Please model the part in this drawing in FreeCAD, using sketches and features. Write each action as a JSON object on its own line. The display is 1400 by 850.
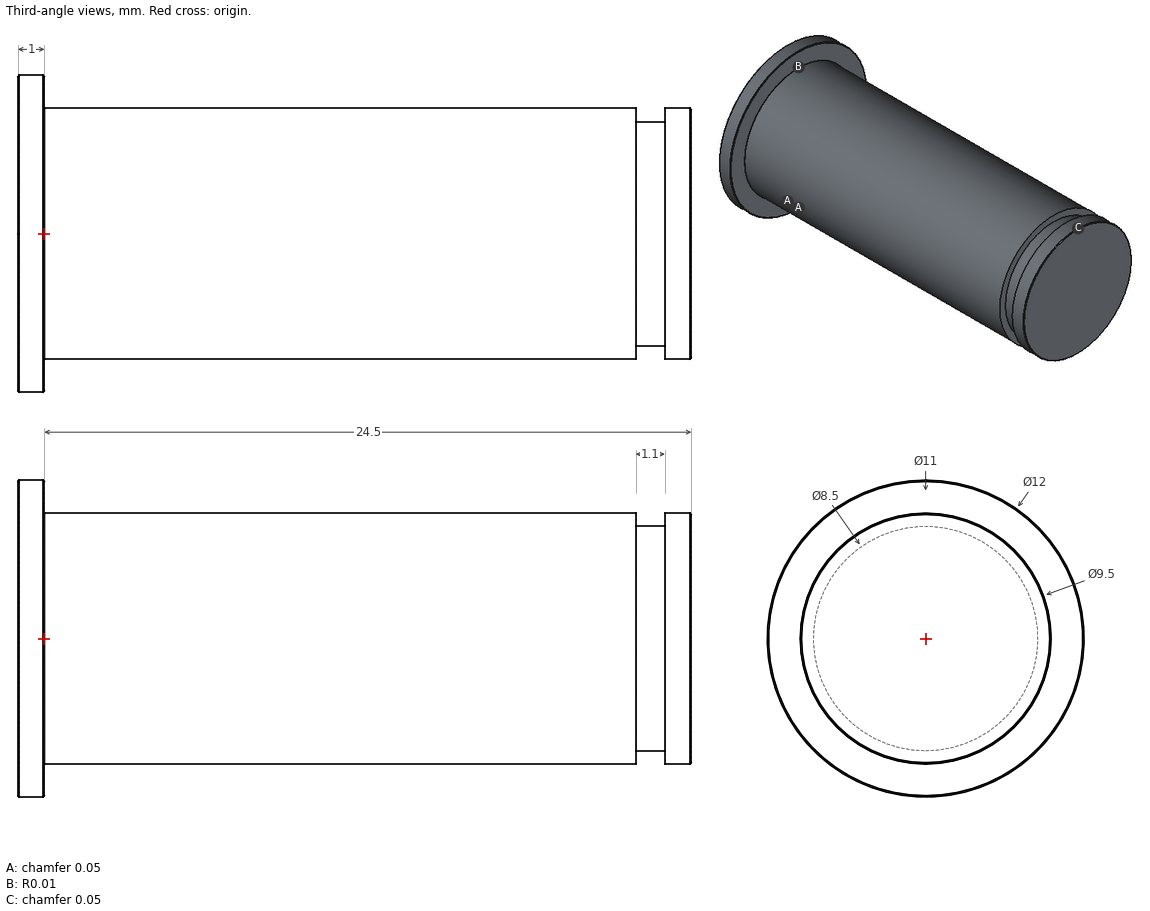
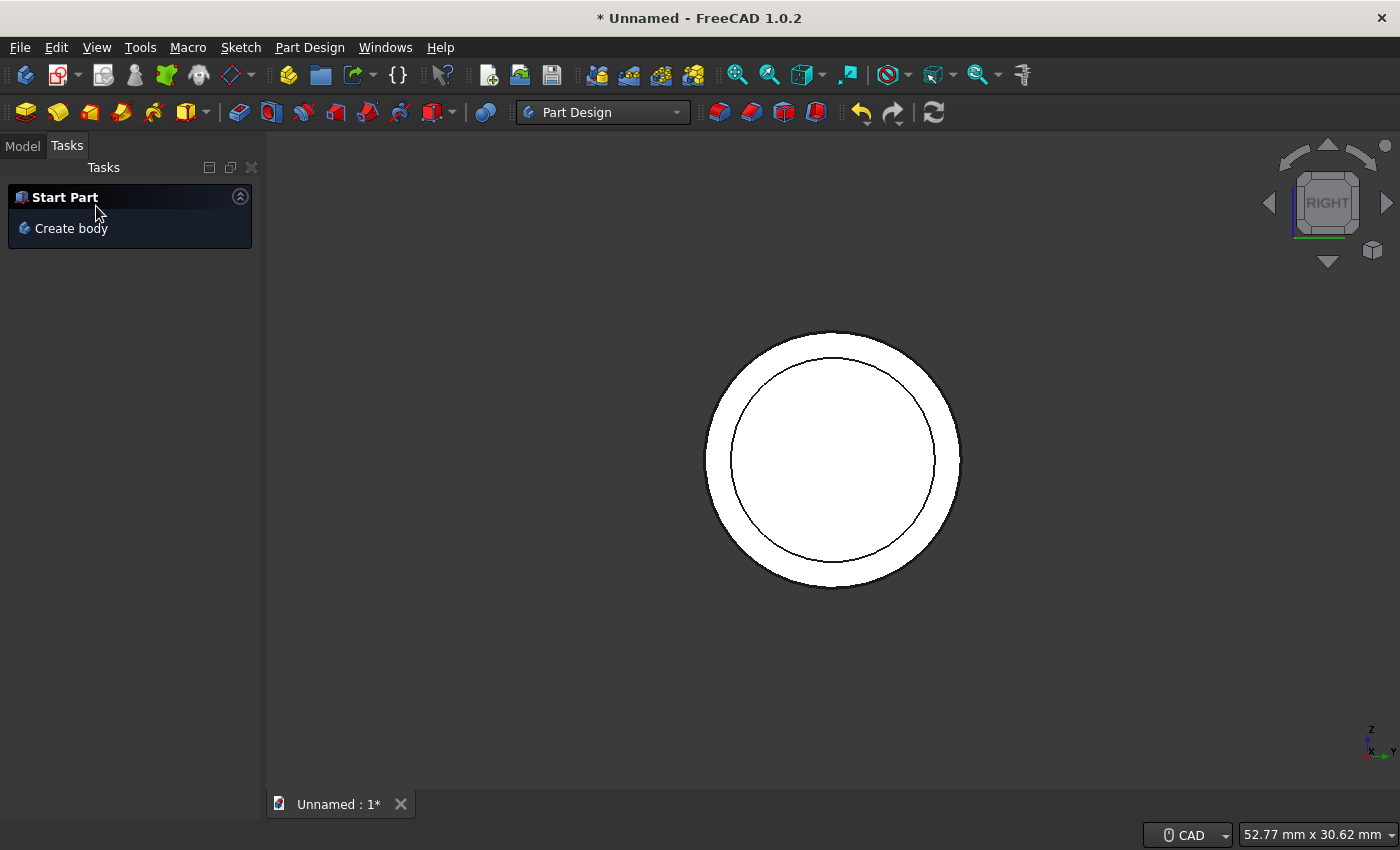
{"action": "key", "text": "v f"}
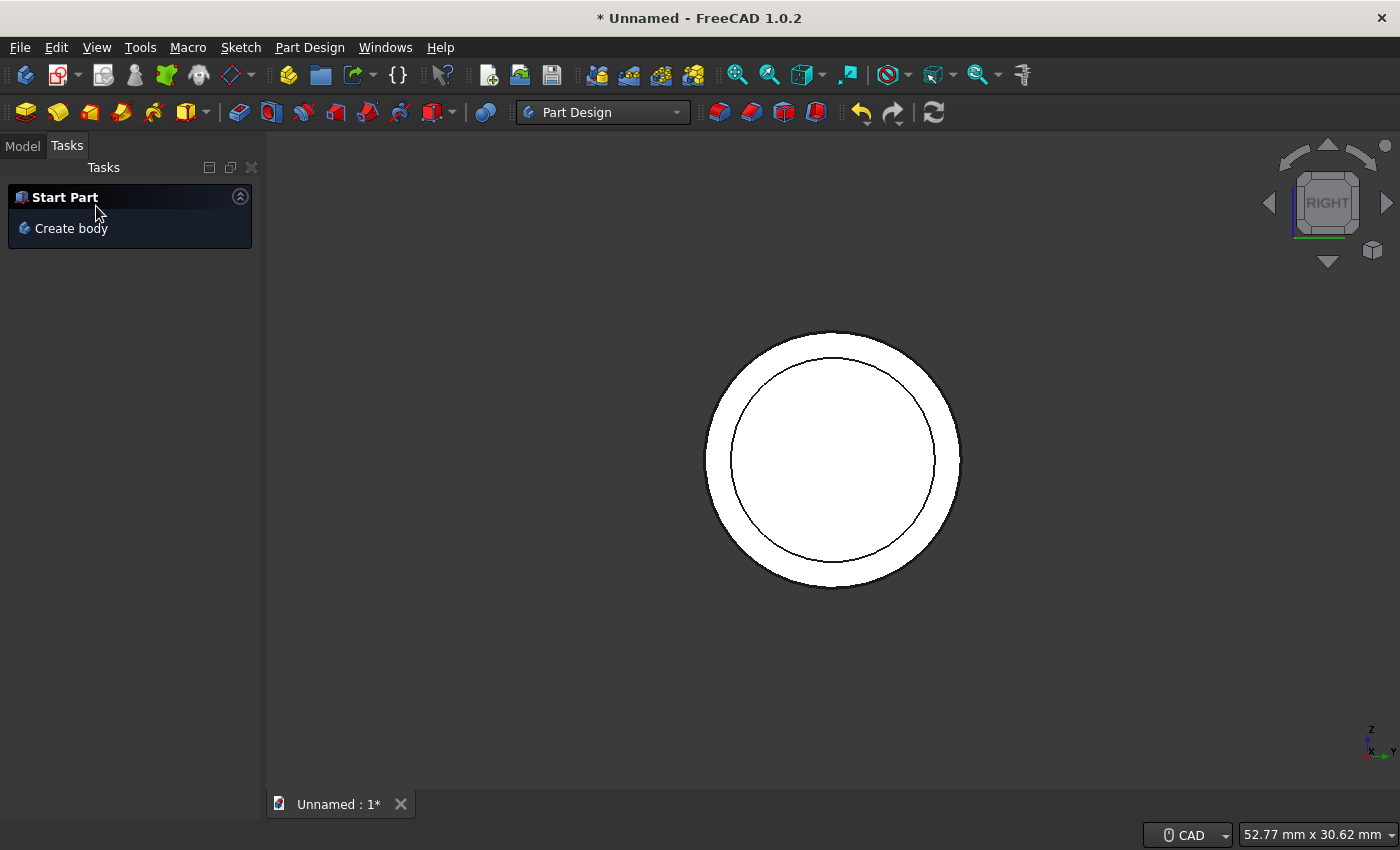
{"action": "key", "text": "5"}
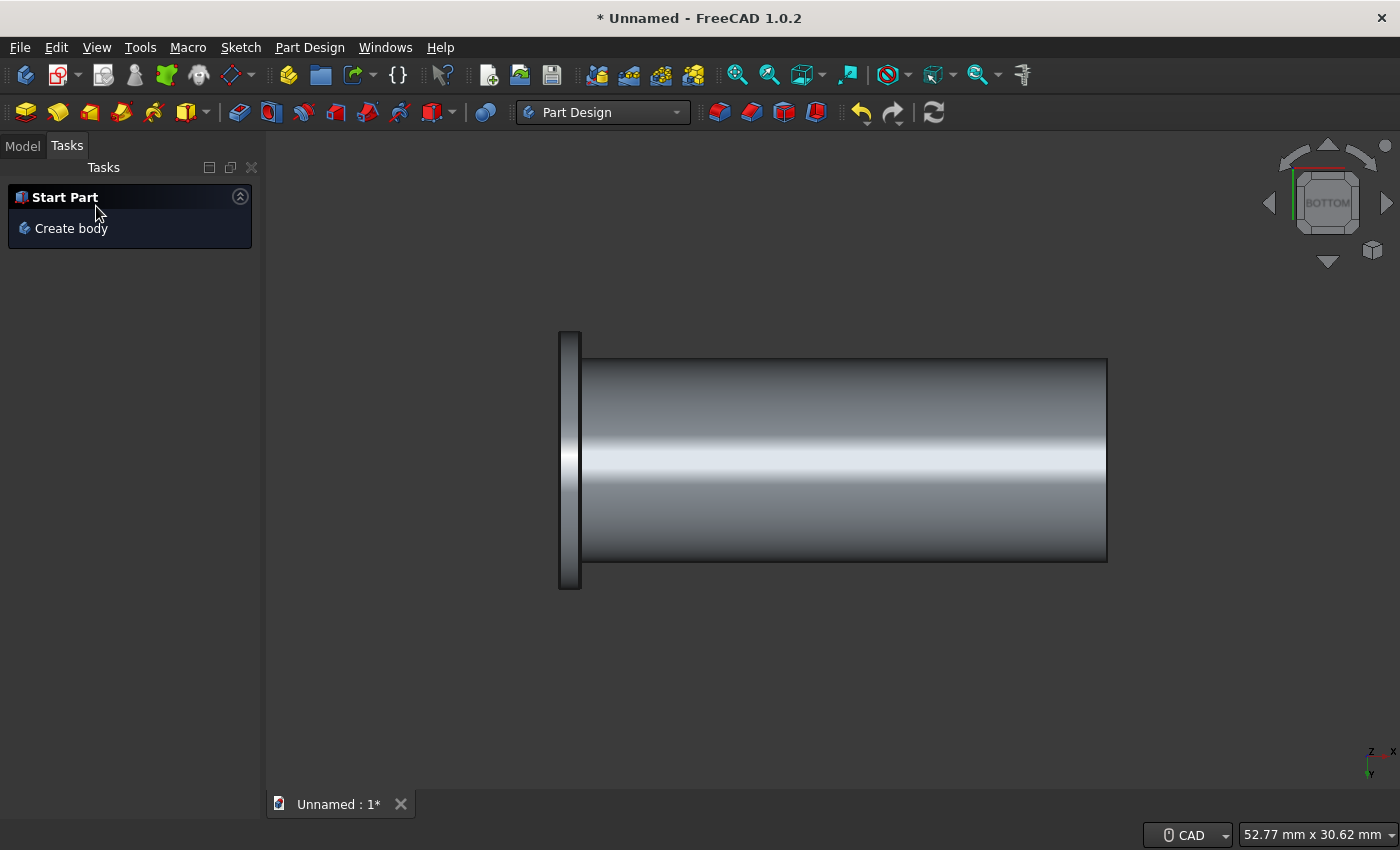
{"action": "key", "text": "4"}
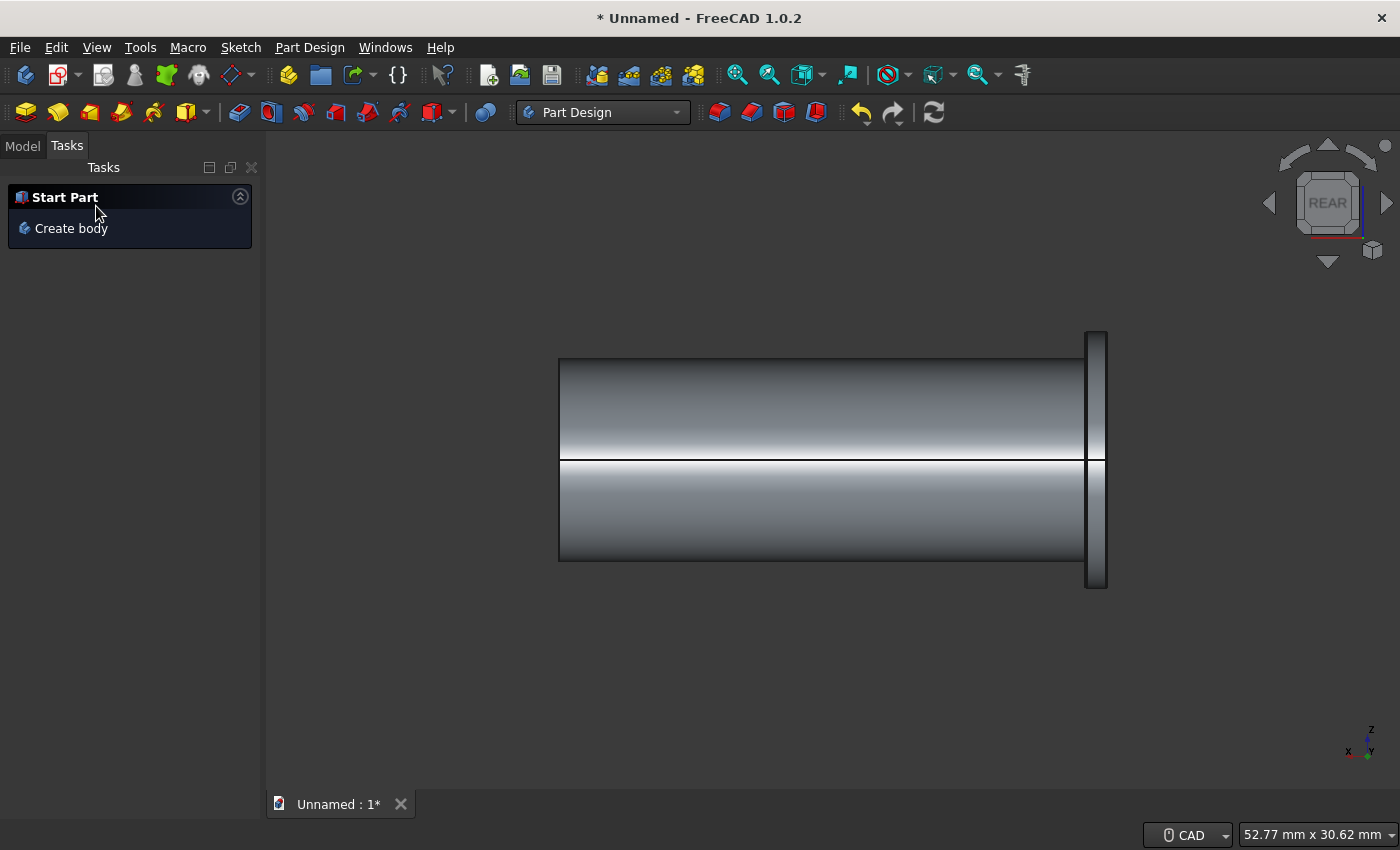
{"action": "key", "text": "6"}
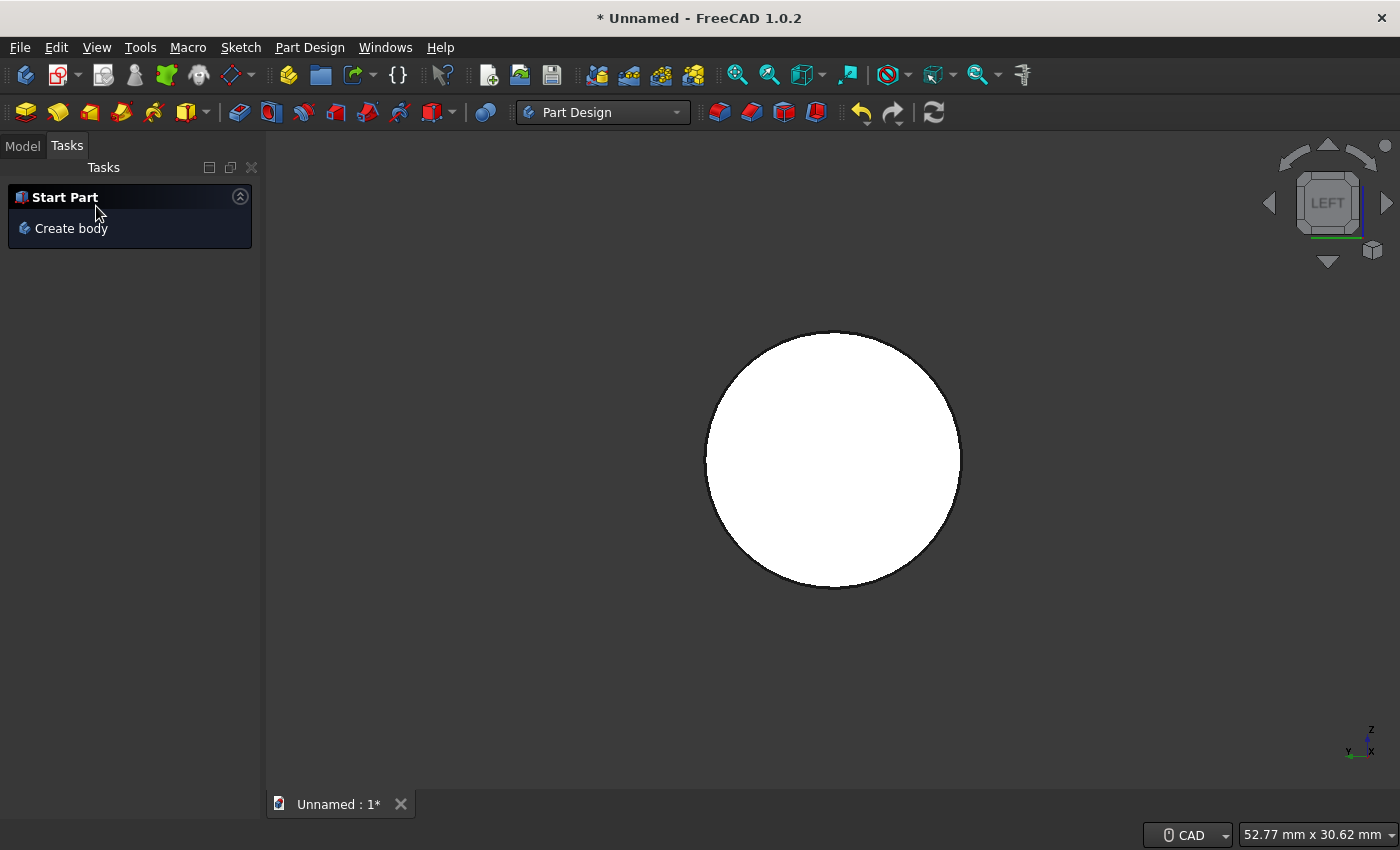
{"action": "key", "text": "v f"}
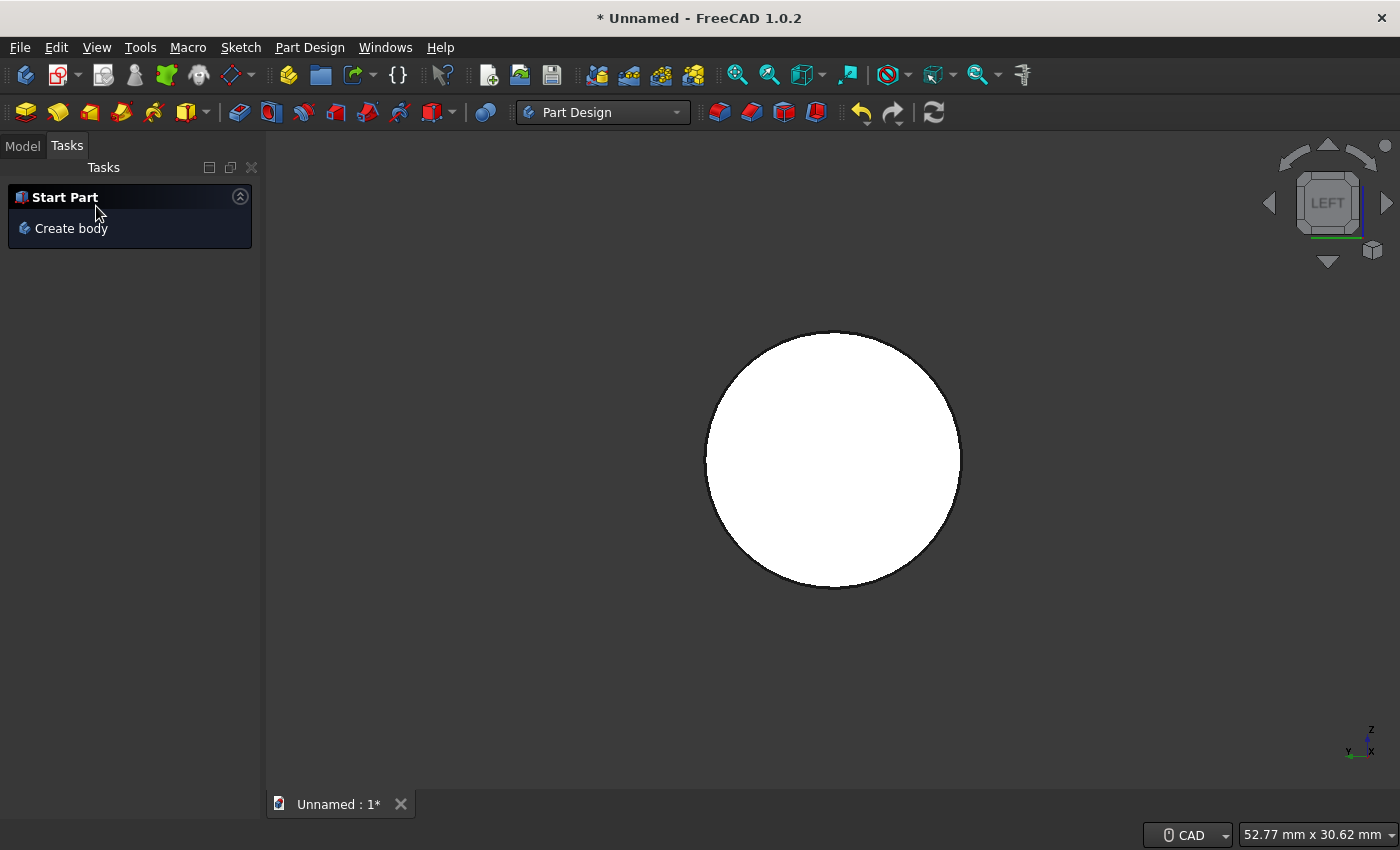
{"action": "key", "text": "v 3"}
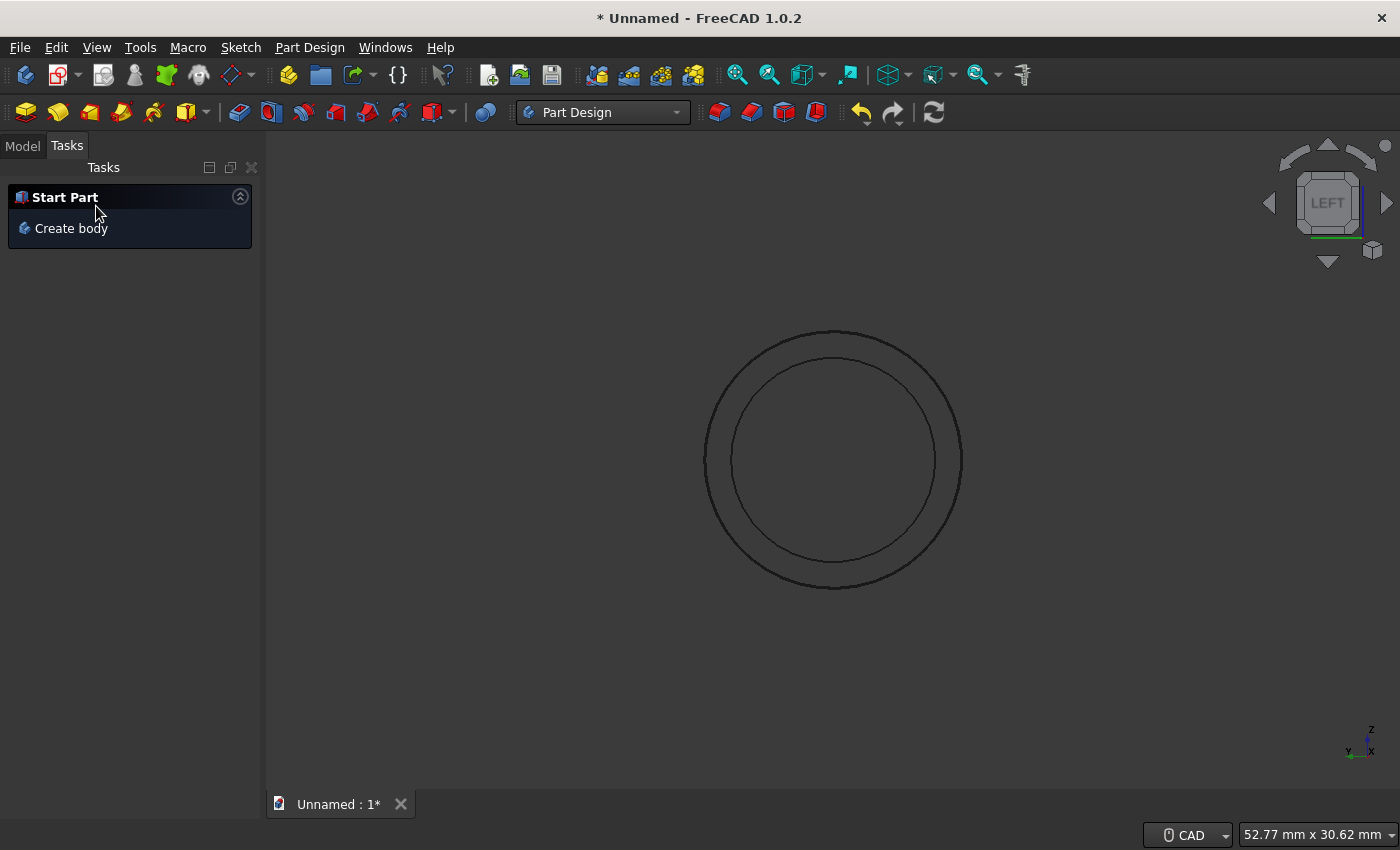
{"action": "key", "text": "0"}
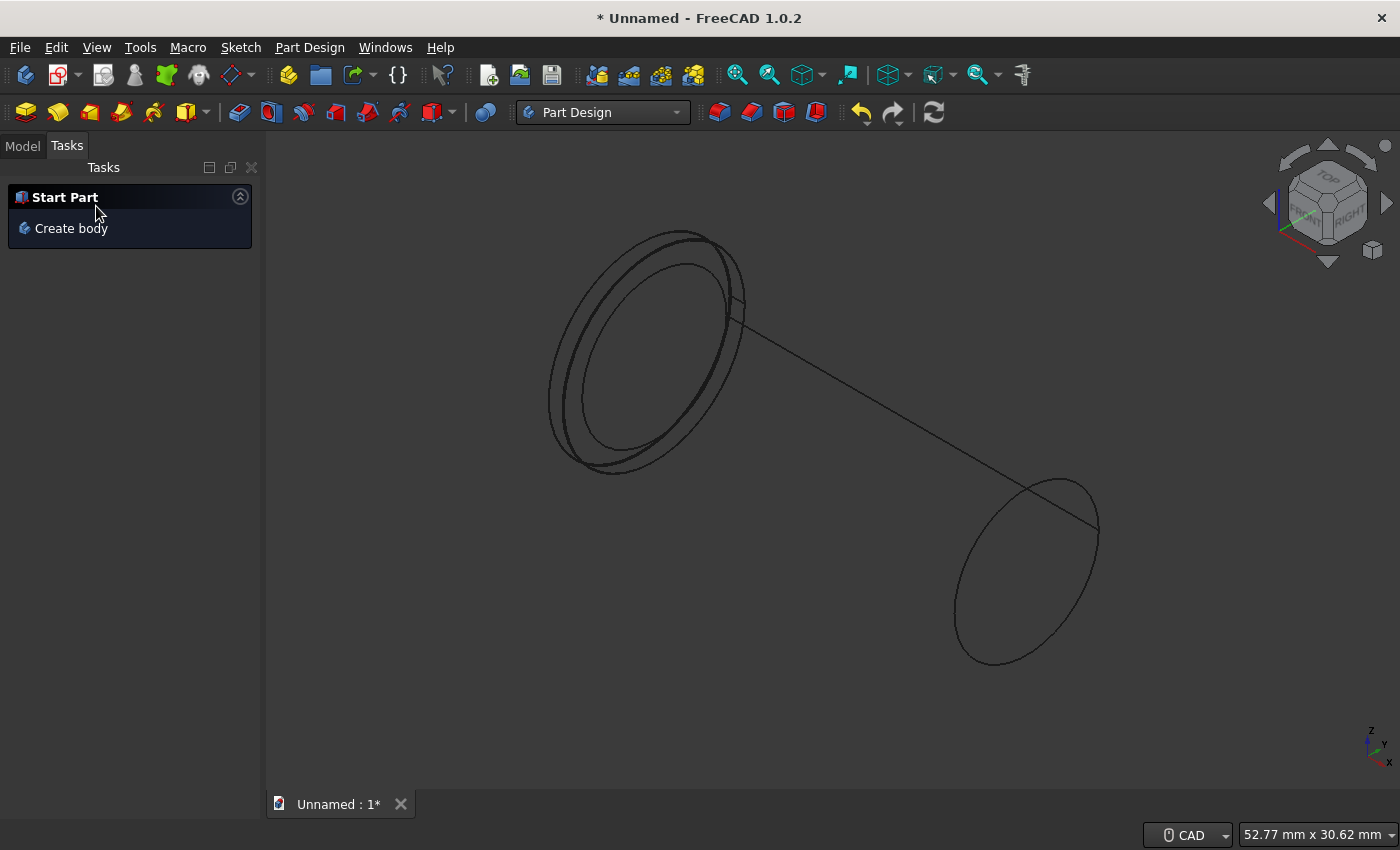
{"action": "left_click", "coordinate": [582, 398]}